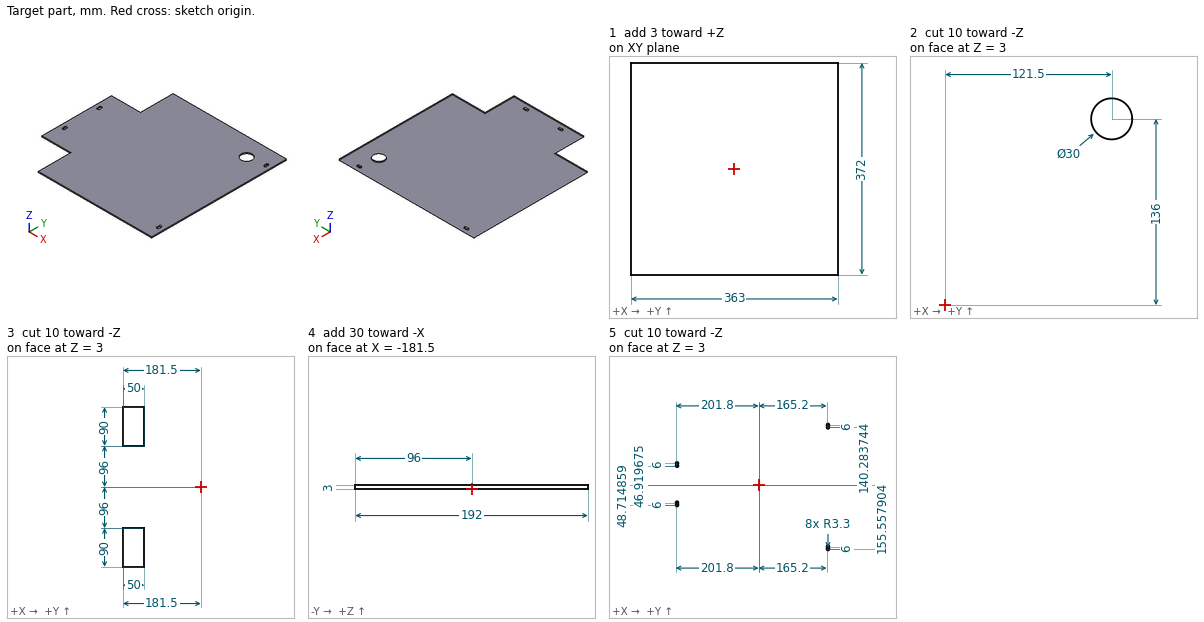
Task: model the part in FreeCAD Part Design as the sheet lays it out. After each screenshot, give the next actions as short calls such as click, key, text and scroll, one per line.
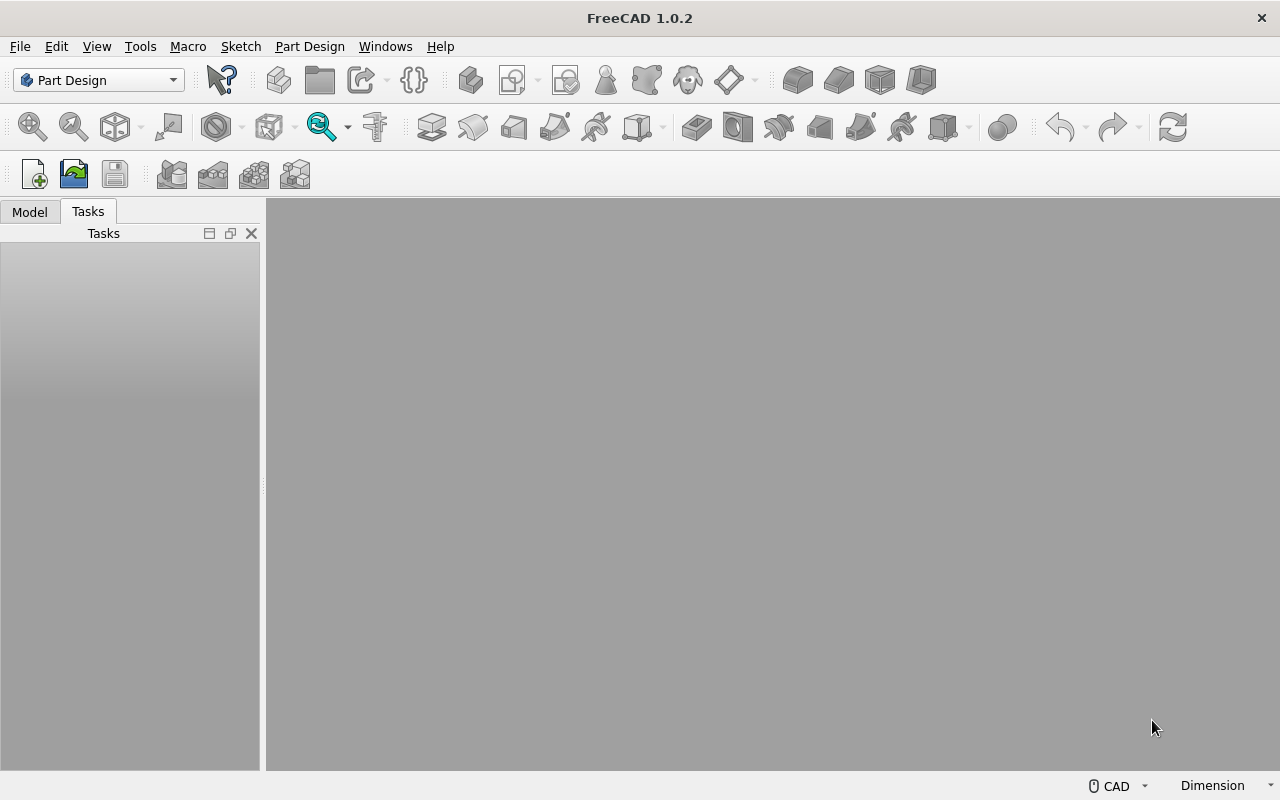
key(ctrl+n)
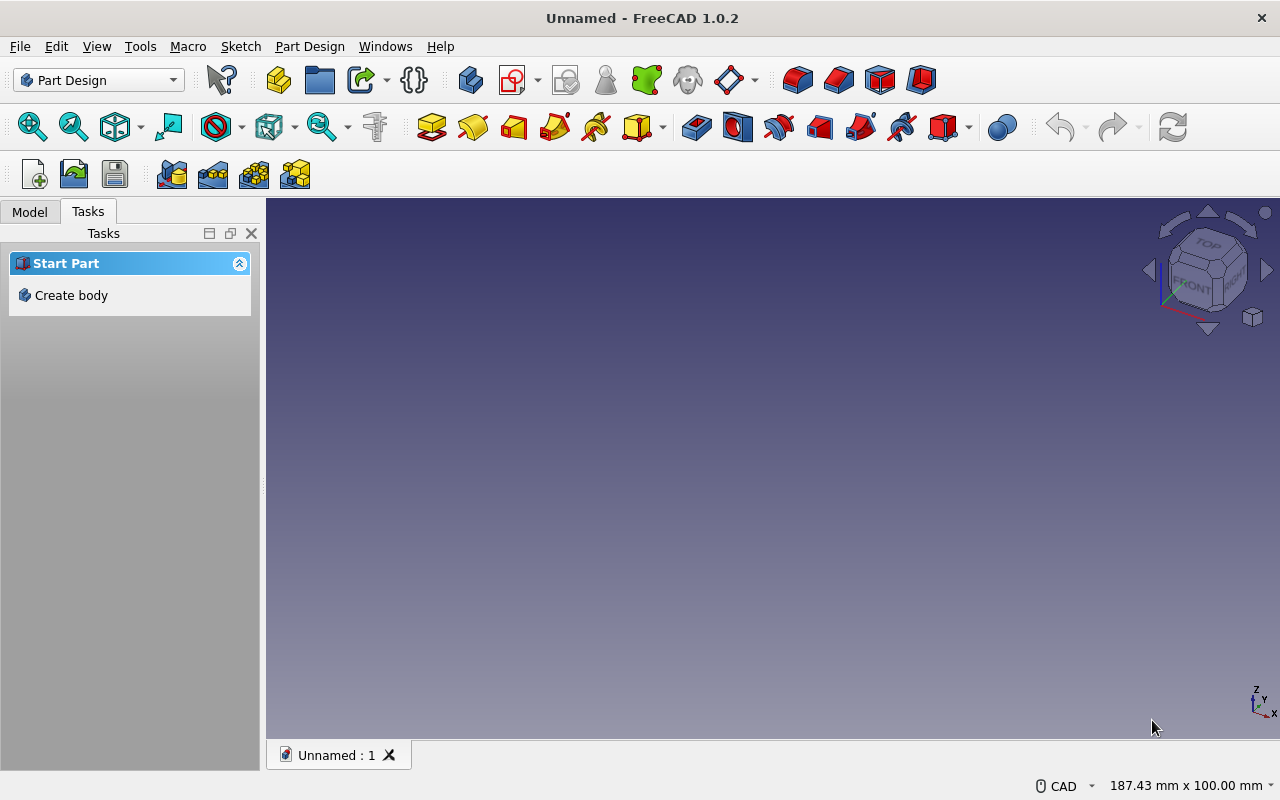
click(512, 80)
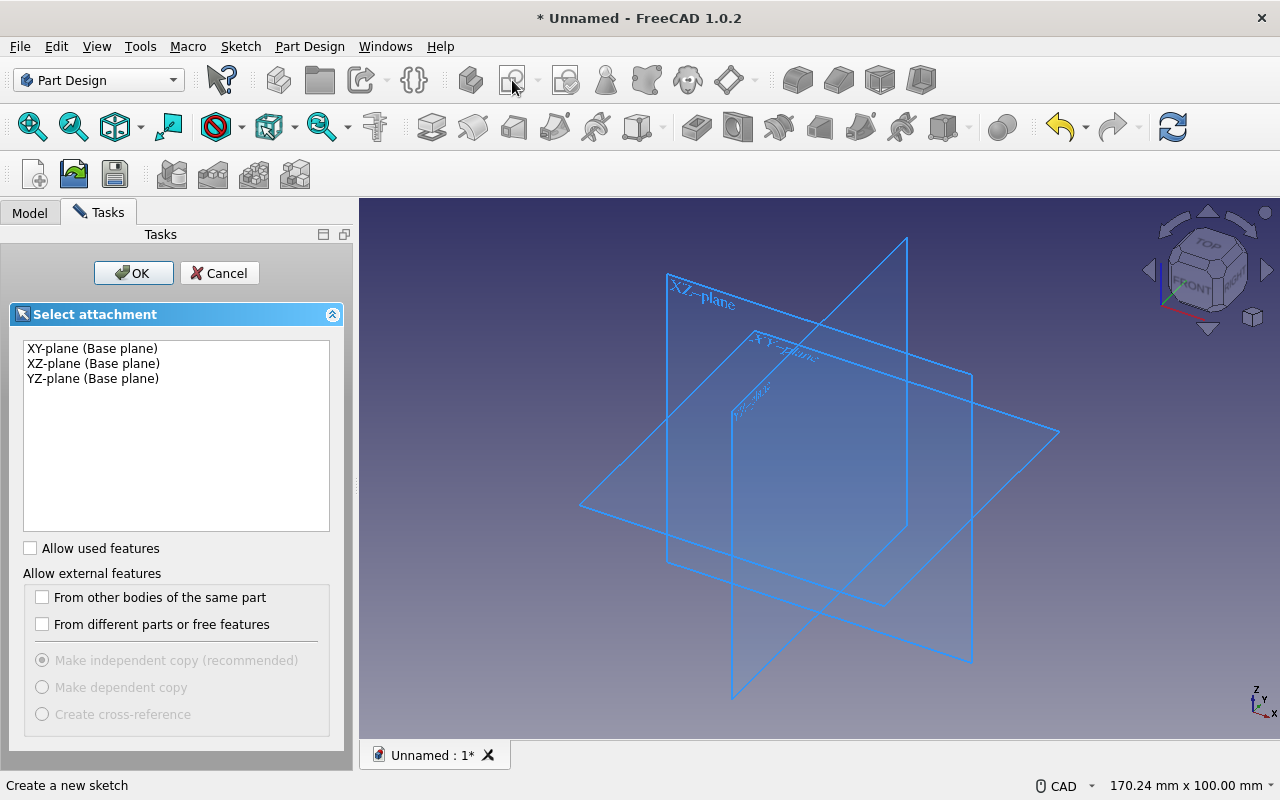
click(84, 348)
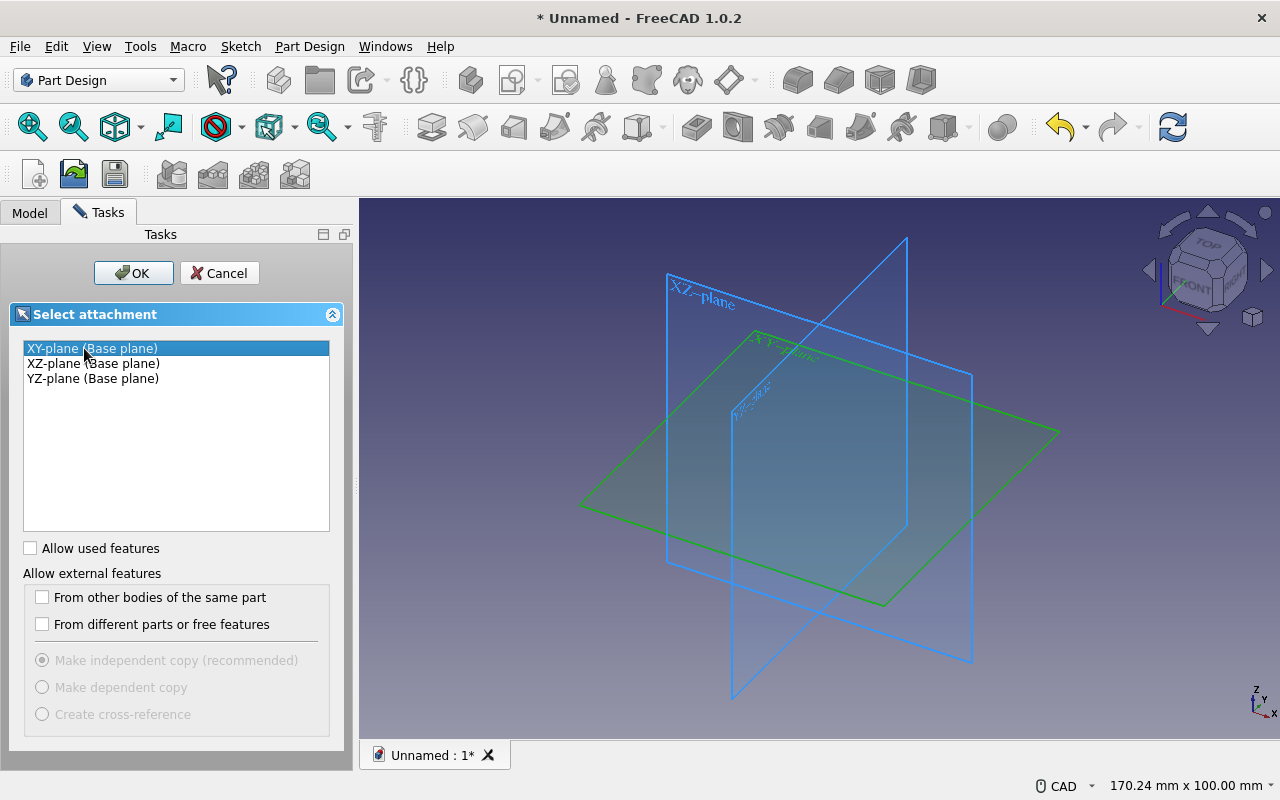
click(134, 273)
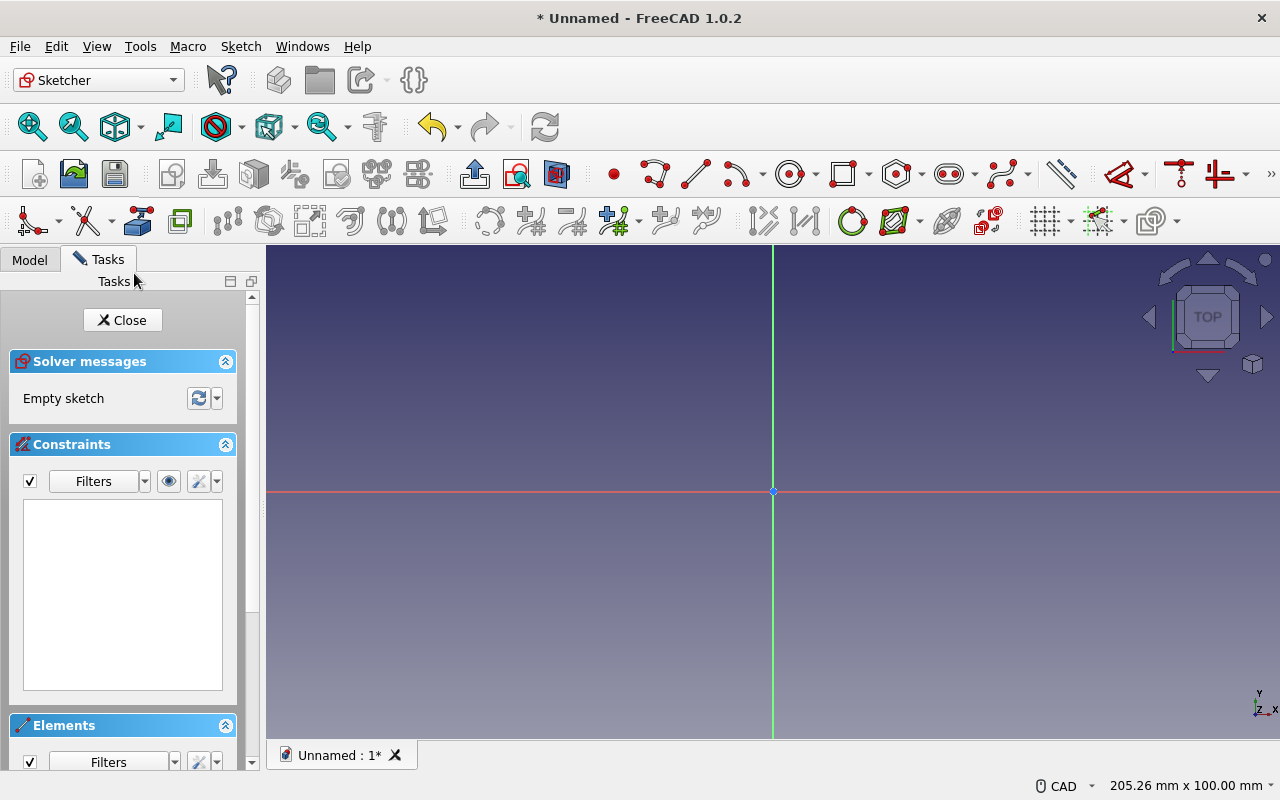
scroll(691, 492, down, 9)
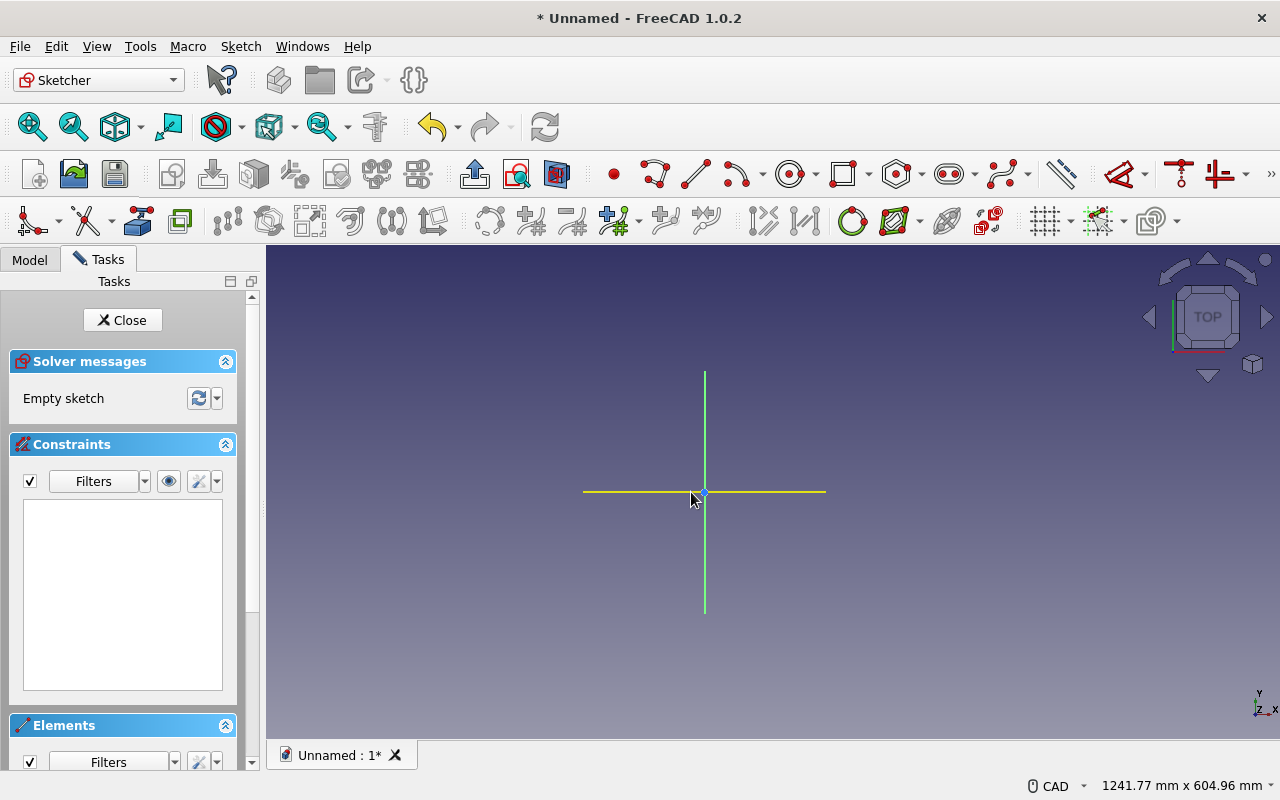
key(g)
key(v)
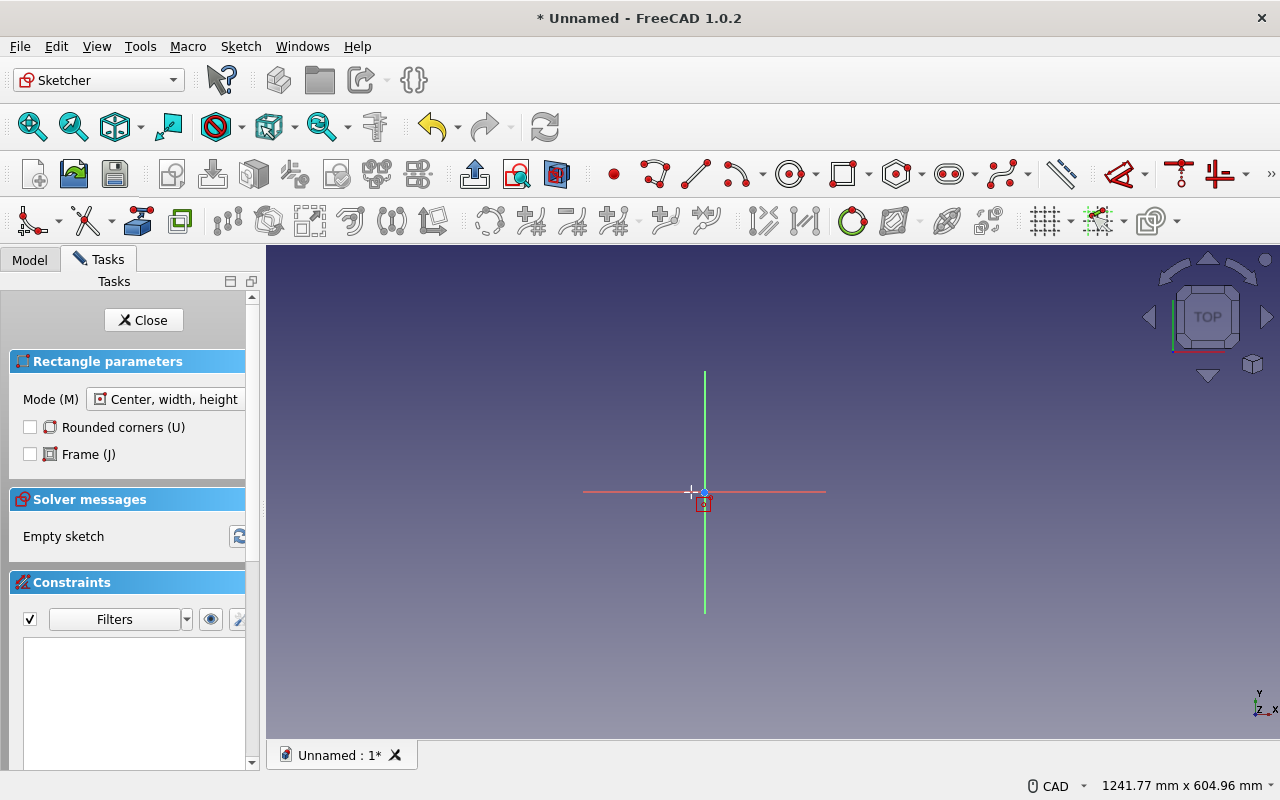
click(705, 492)
move(853, 341)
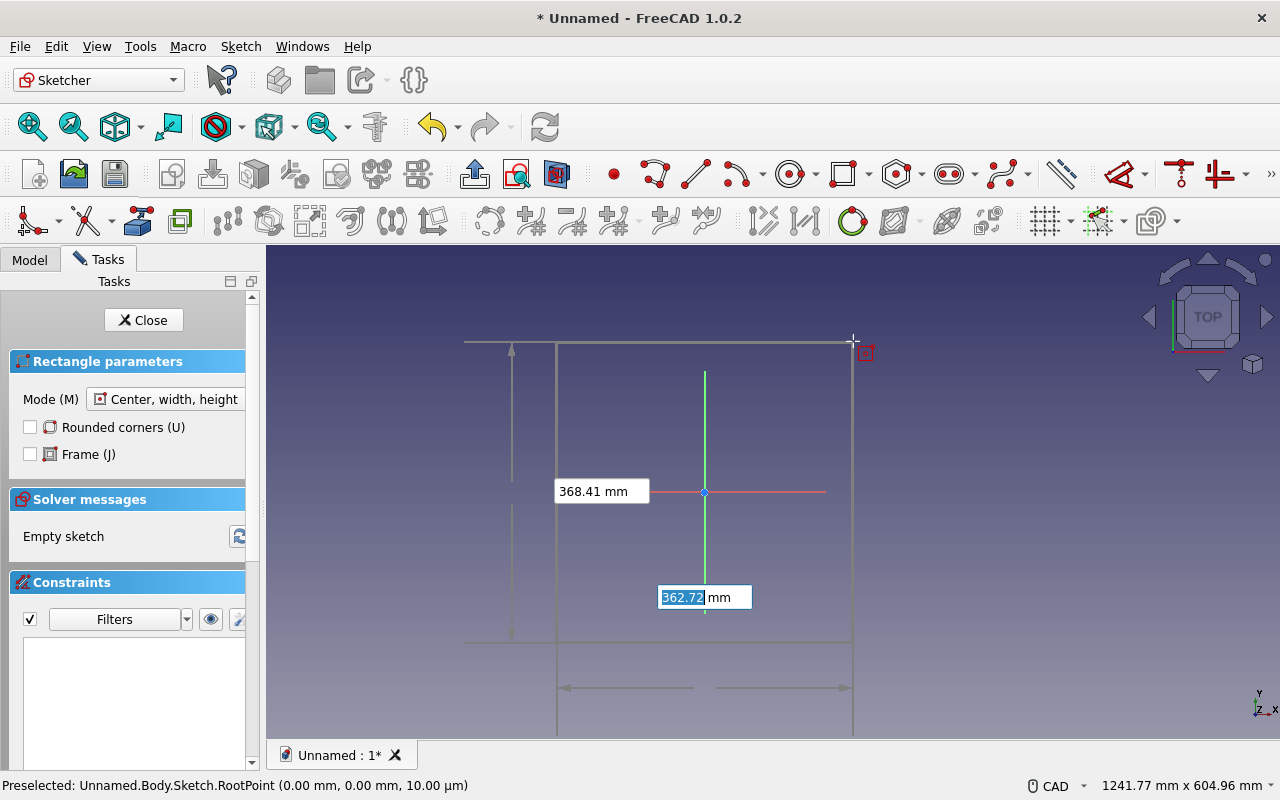
text(363)
key(Tab)
text(372)
key(Return)
key(Escape)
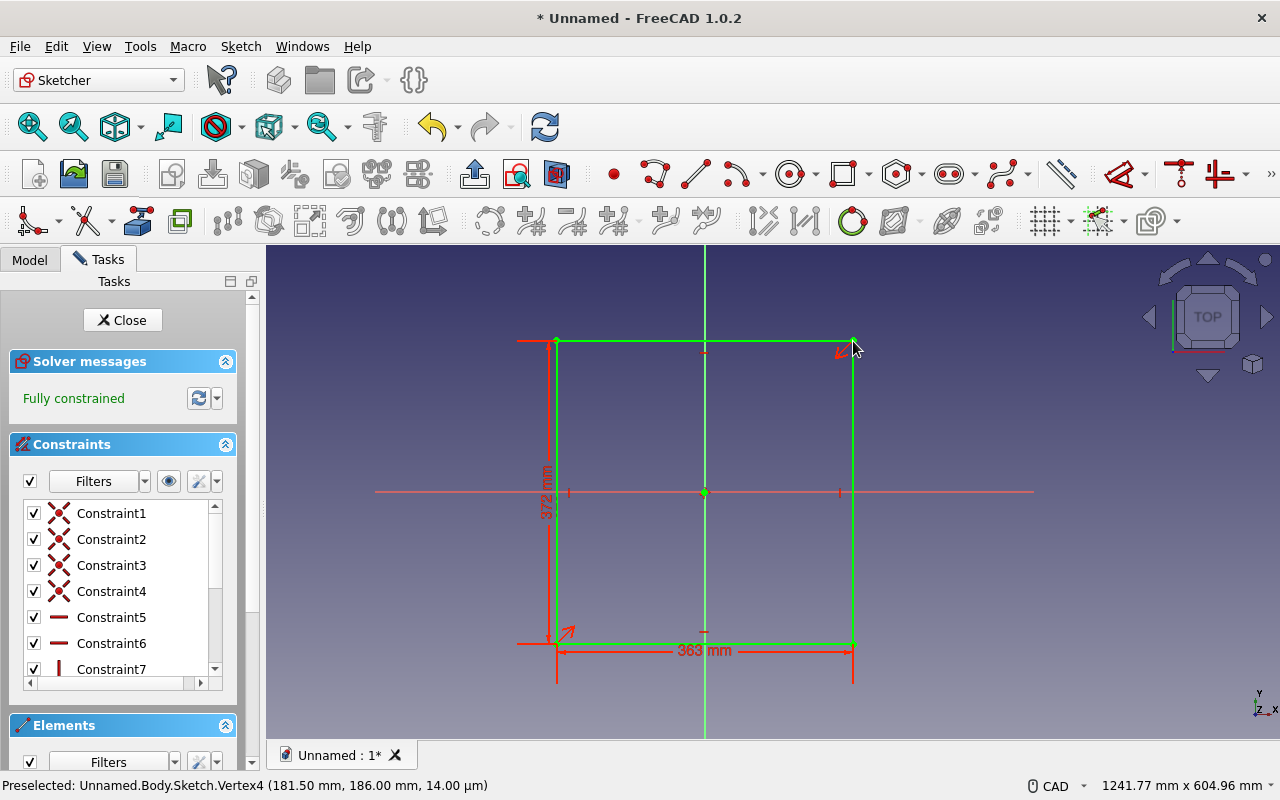
click(123, 320)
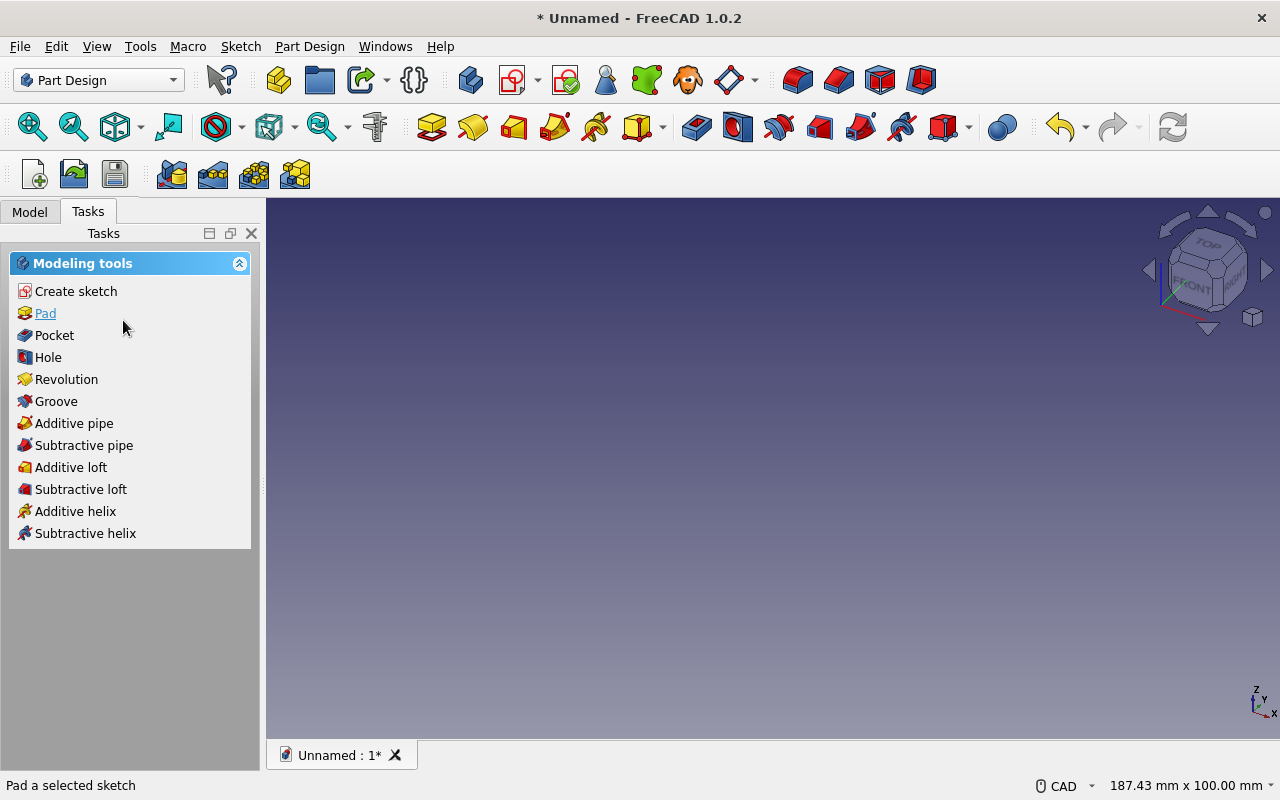
click(432, 128)